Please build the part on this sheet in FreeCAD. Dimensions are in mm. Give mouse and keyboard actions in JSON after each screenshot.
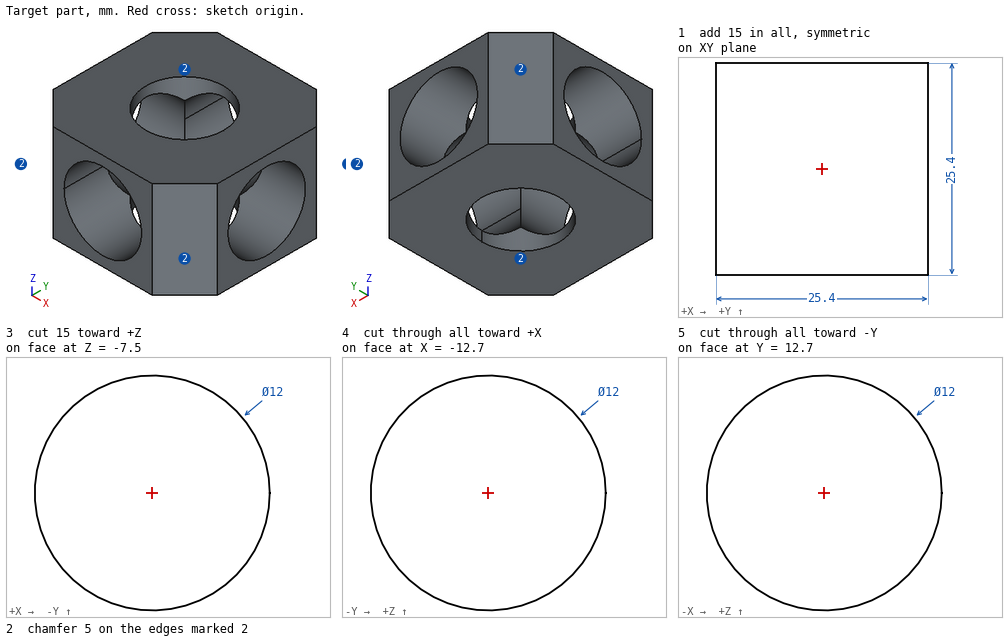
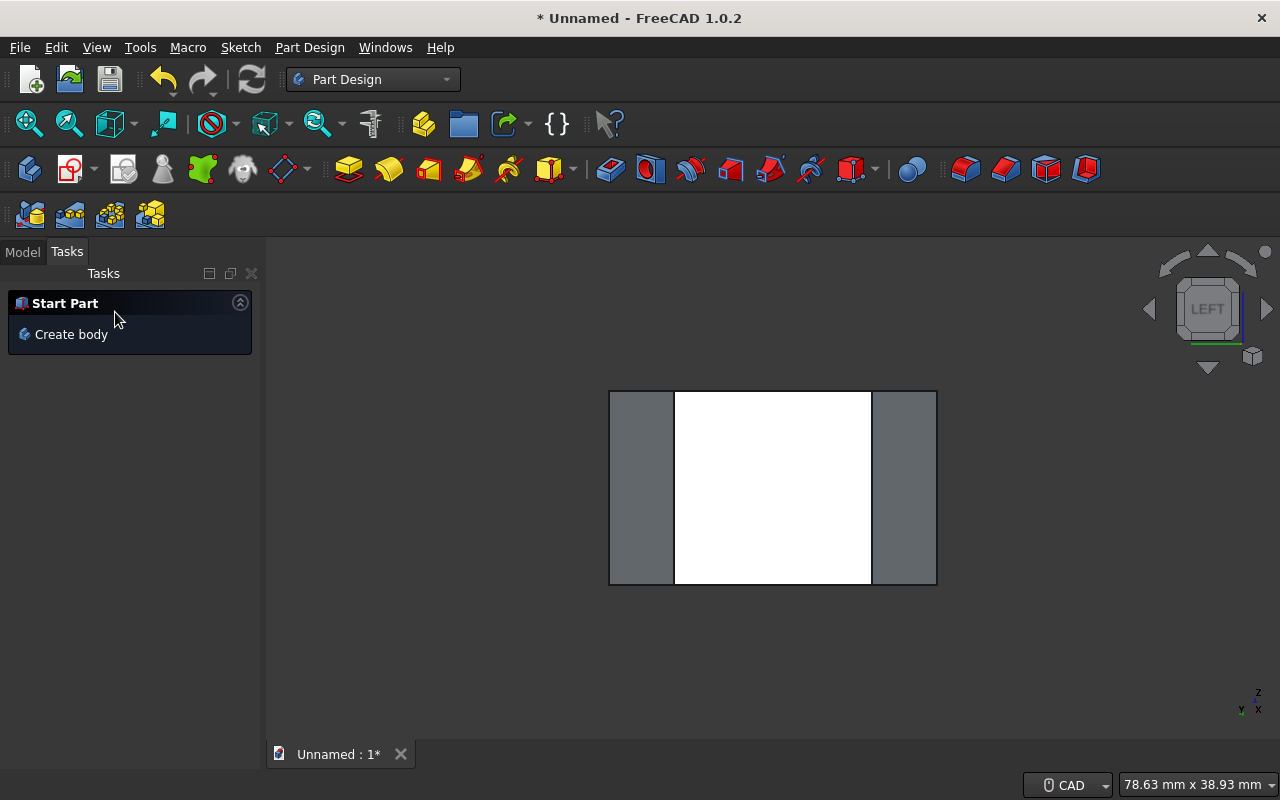
{"action": "left_click", "coordinate": [773, 487]}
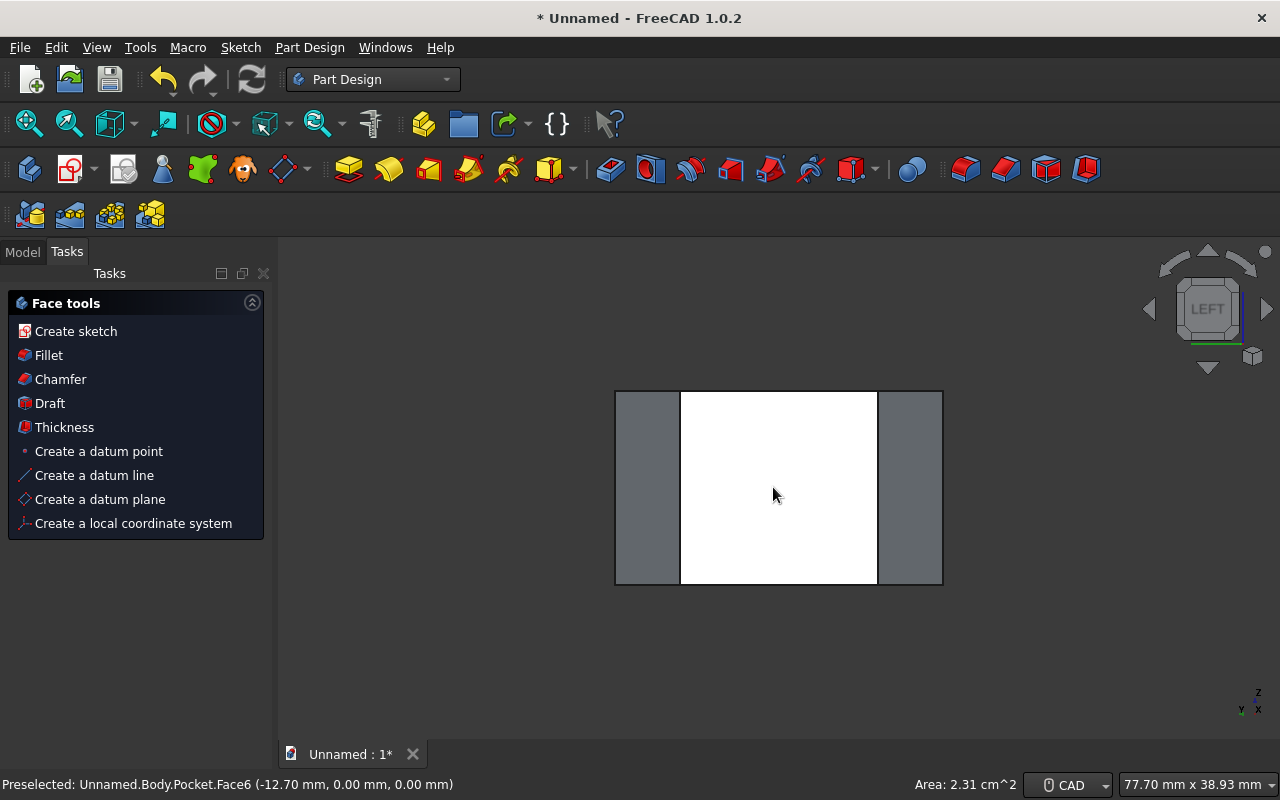
{"action": "left_click", "coordinate": [70, 170]}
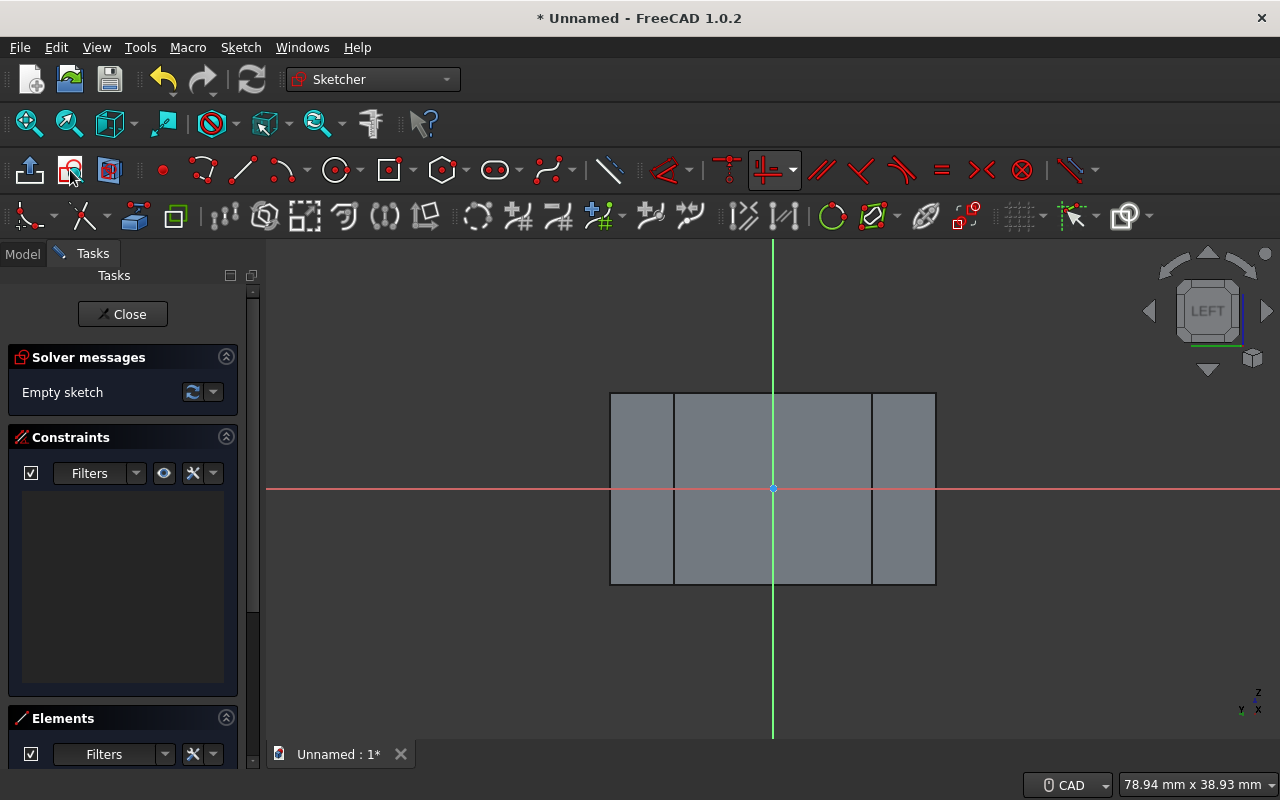
{"action": "scroll", "coordinate": [829, 489], "scroll_direction": "up", "scroll_amount": 4}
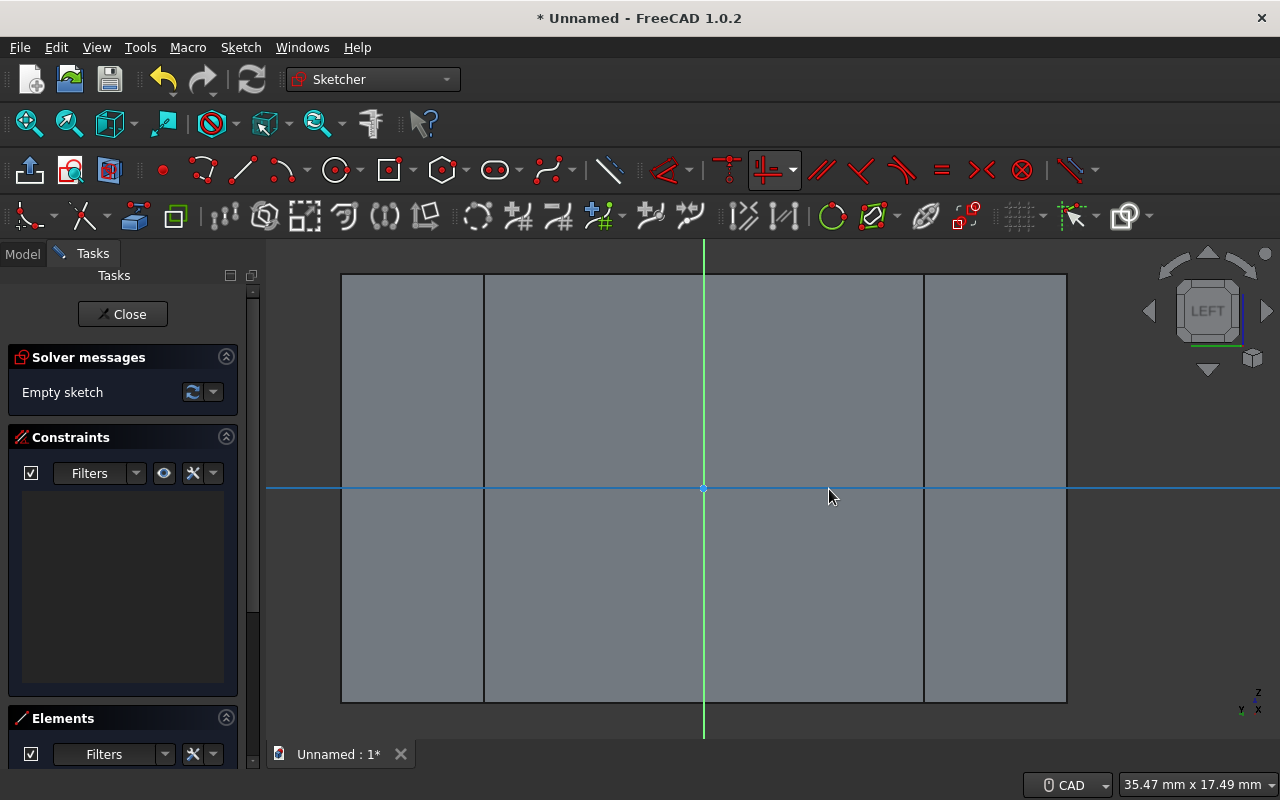
{"action": "key", "text": "g c"}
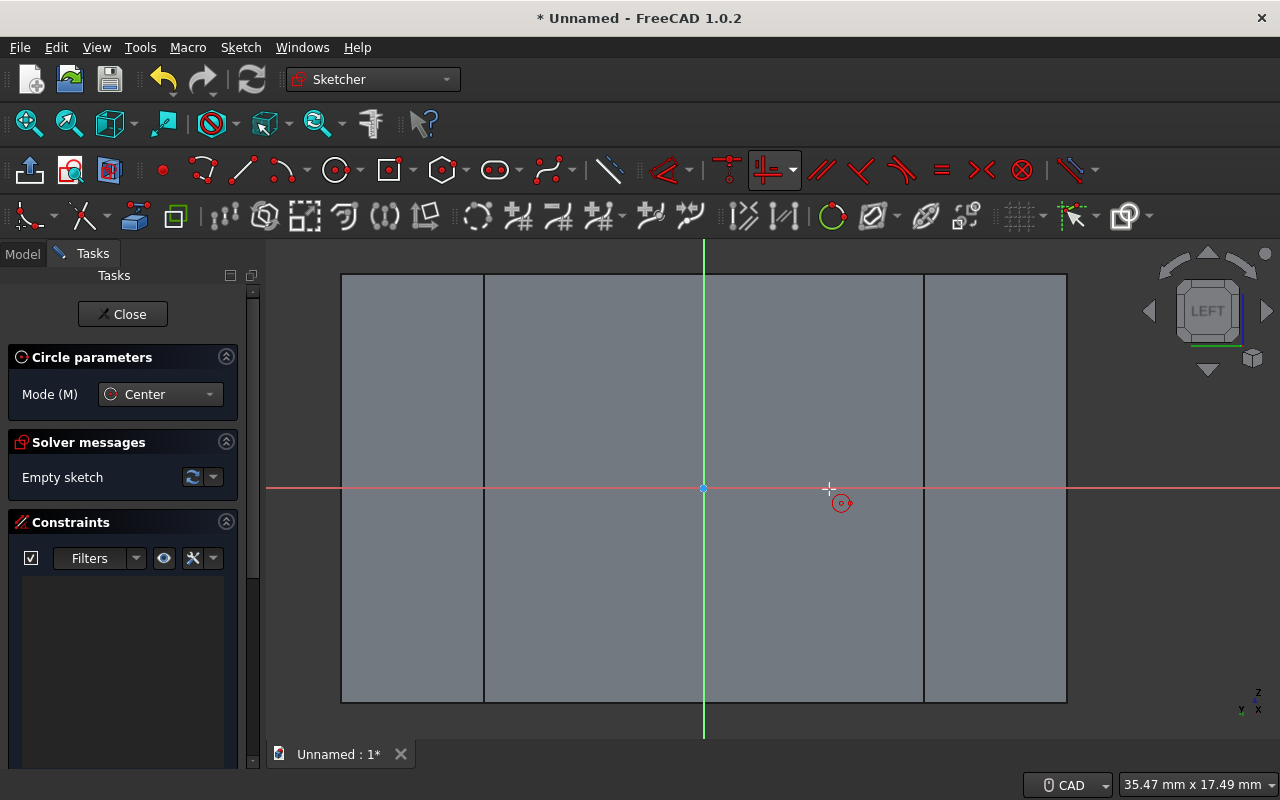
{"action": "left_click", "coordinate": [704, 488]}
{"action": "left_click", "coordinate": [825, 367]}
{"action": "key", "text": "Escape"}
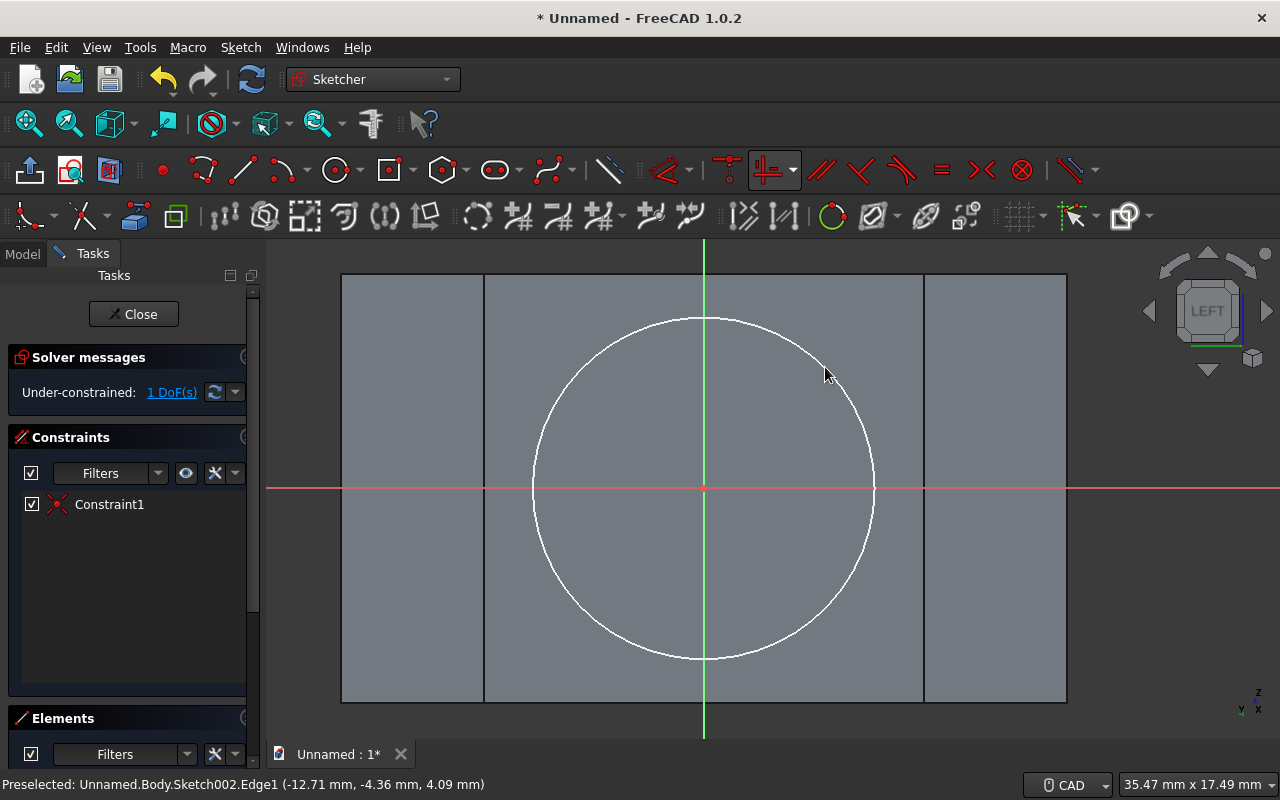
{"action": "key", "text": "d"}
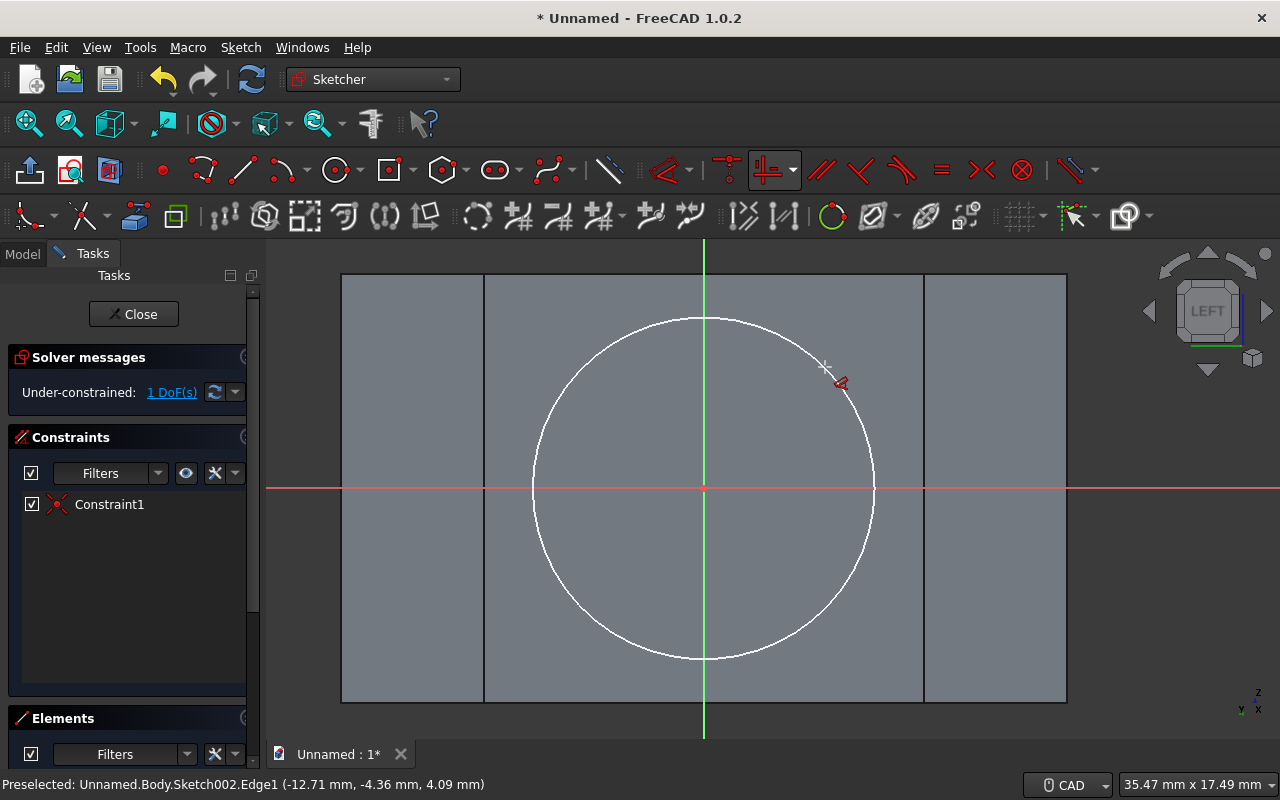
{"action": "left_click", "coordinate": [824, 367]}
{"action": "left_click", "coordinate": [847, 344]}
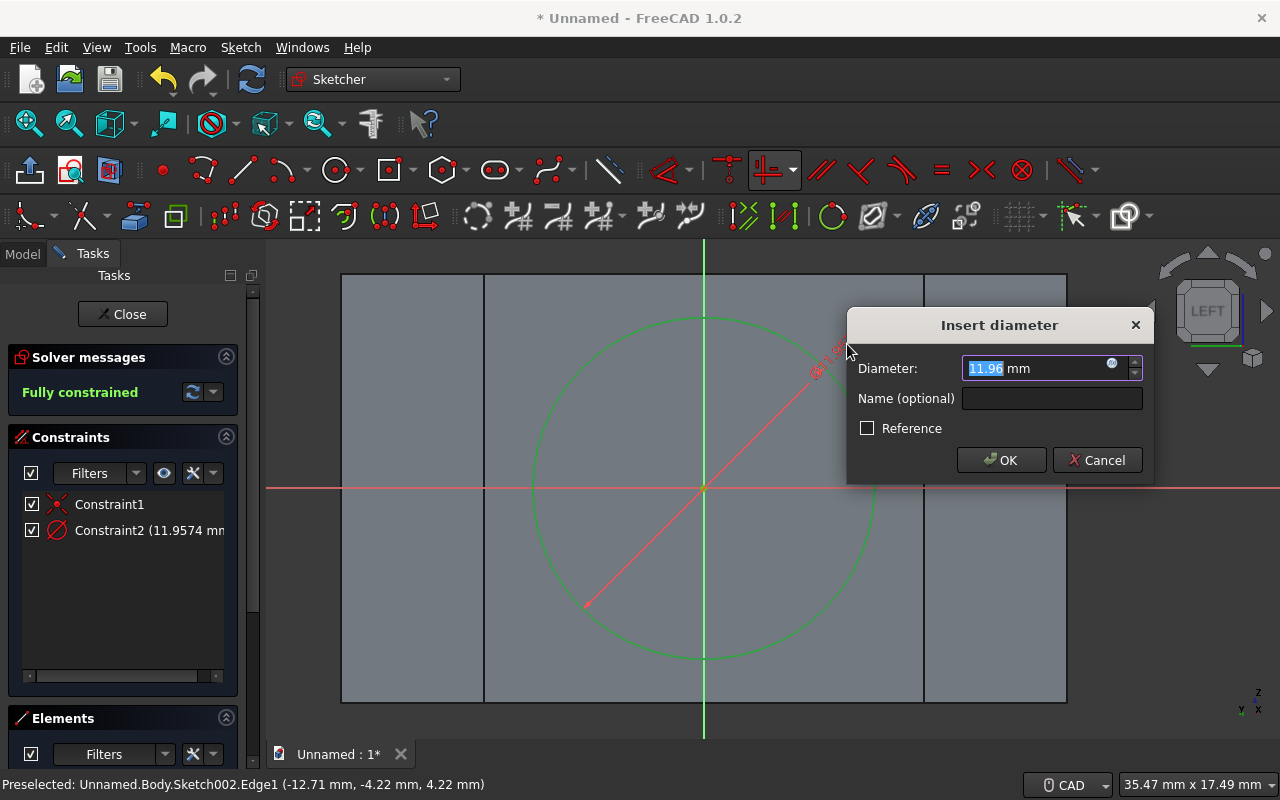
{"action": "type", "text": "12"}
{"action": "key", "text": "Return"}
{"action": "key", "text": "Escape"}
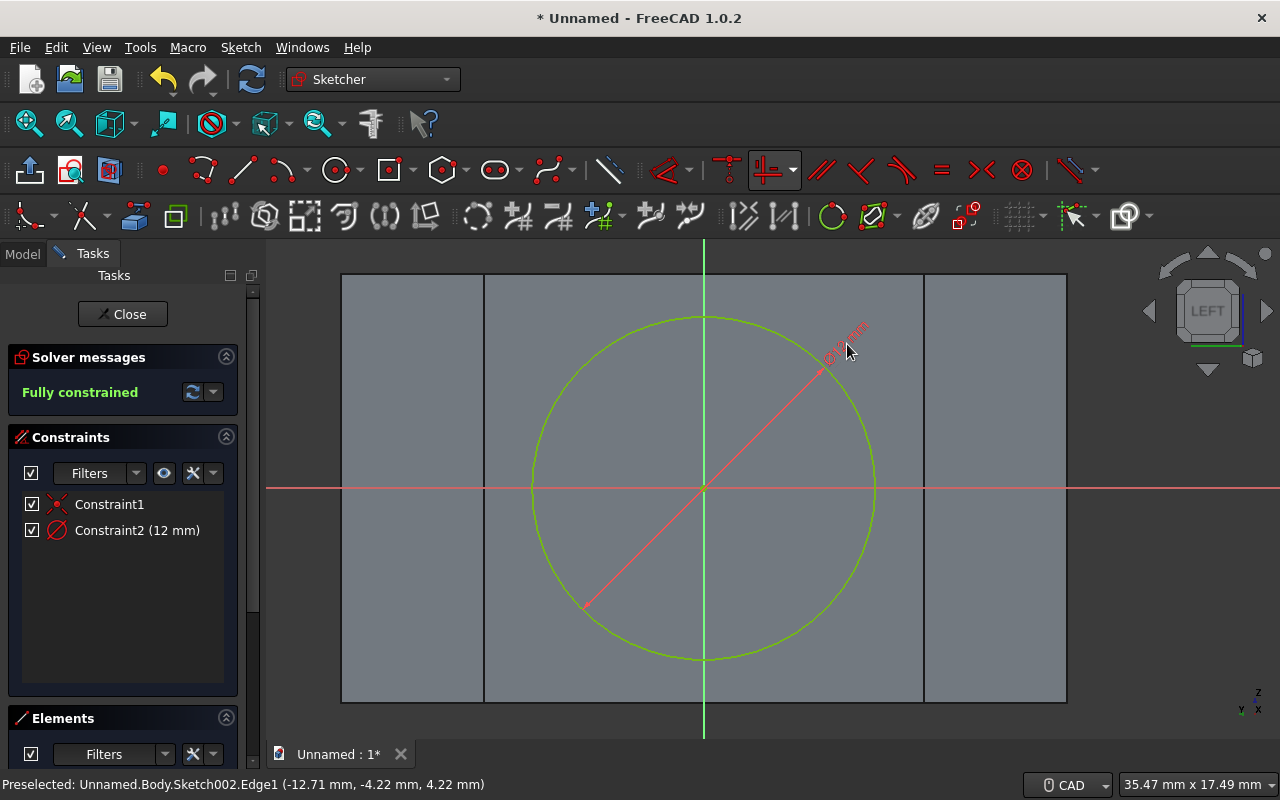
{"action": "left_click", "coordinate": [123, 314]}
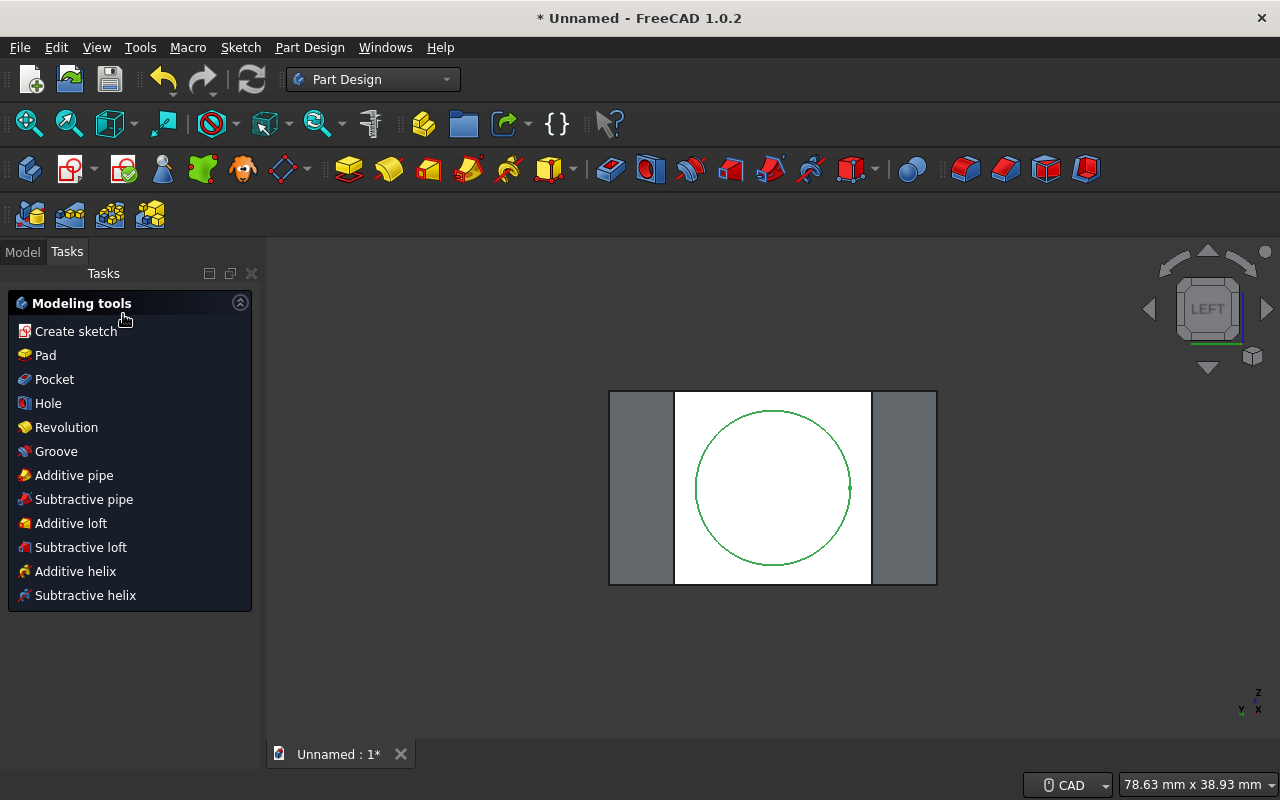
{"action": "left_click", "coordinate": [612, 170]}